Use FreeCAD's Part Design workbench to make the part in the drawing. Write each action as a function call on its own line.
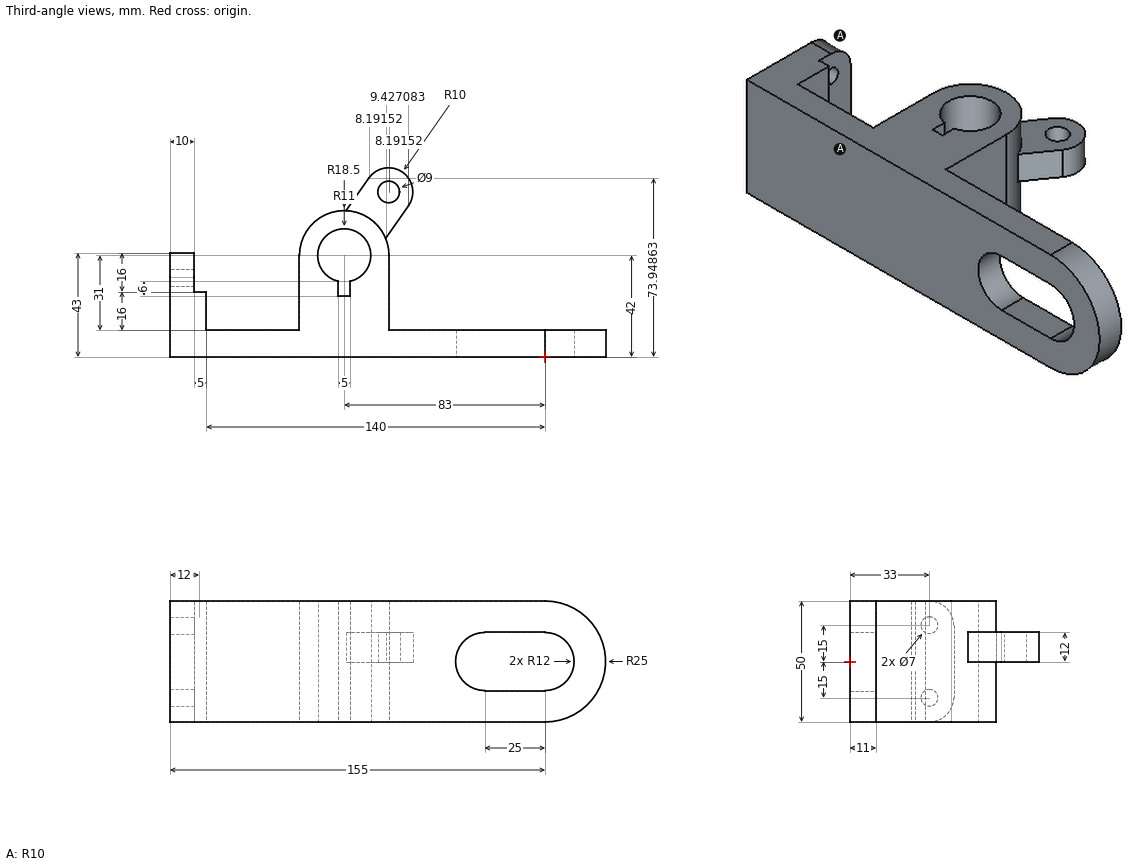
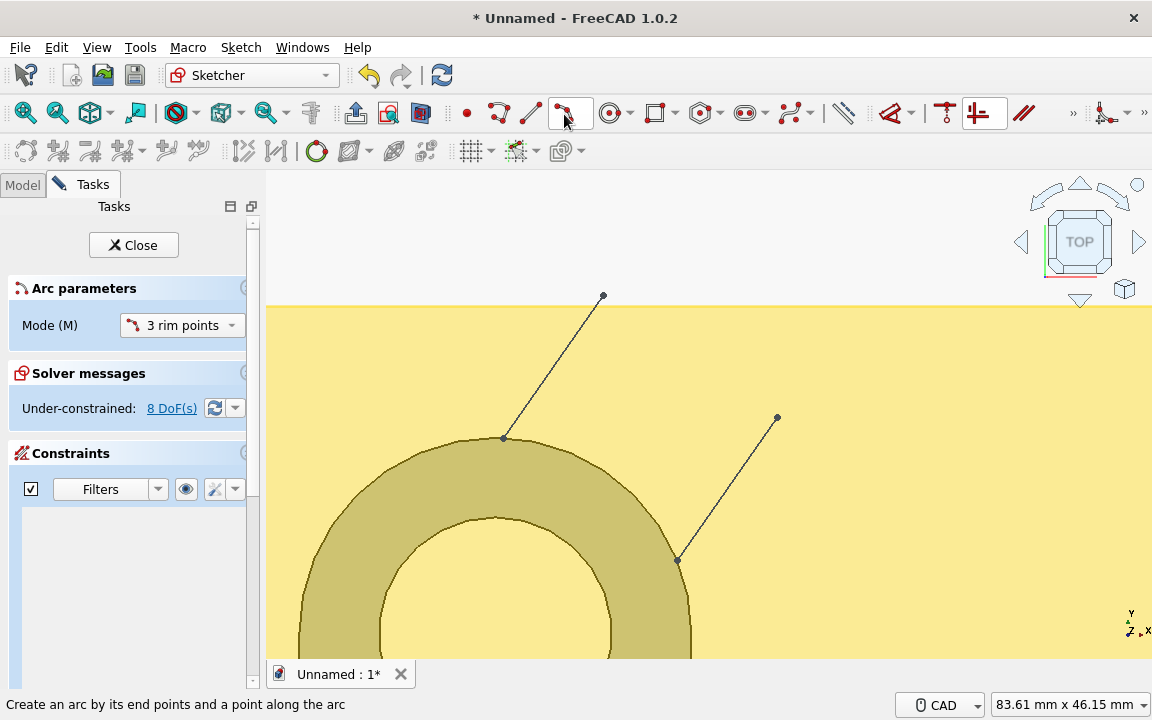
click(777, 418)
click(603, 296)
click(751, 269)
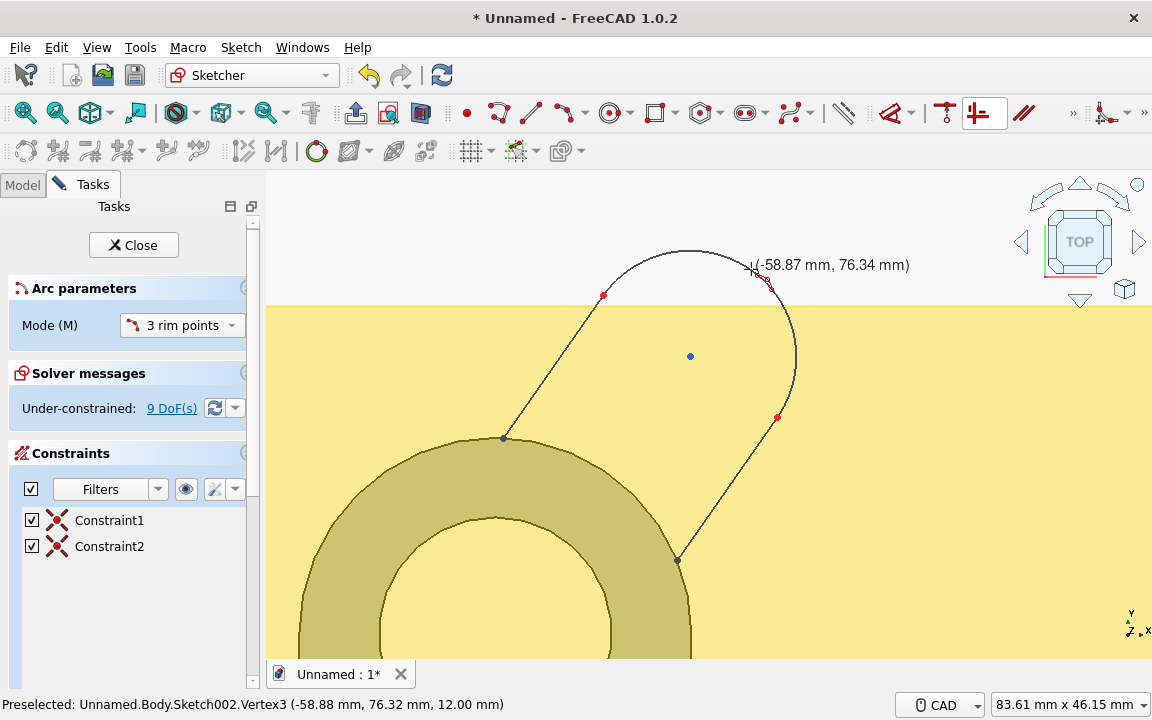
click(503, 439)
click(677, 561)
click(608, 473)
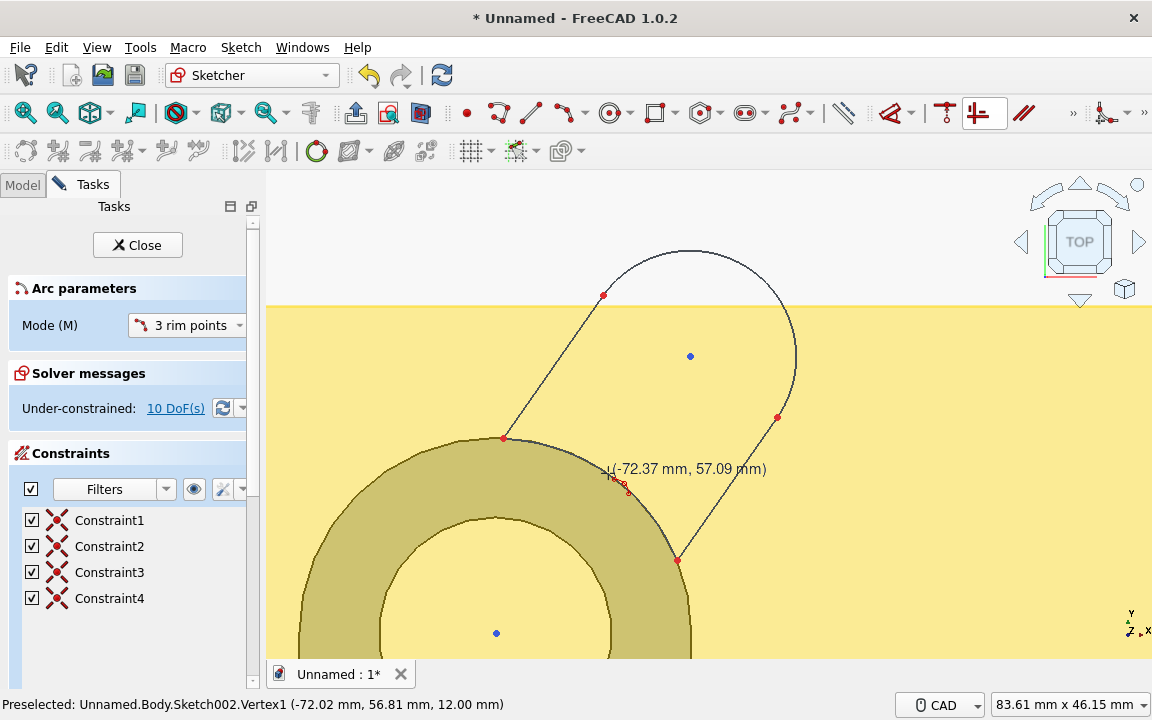
click(610, 114)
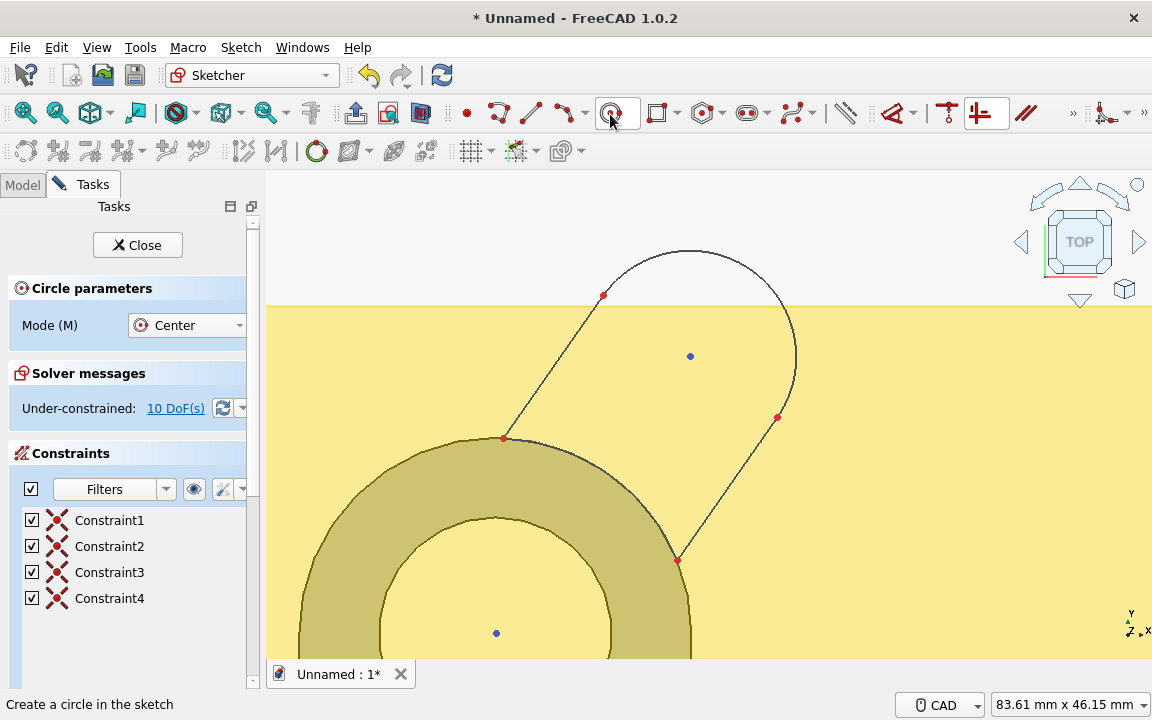
click(690, 356)
move(724, 322)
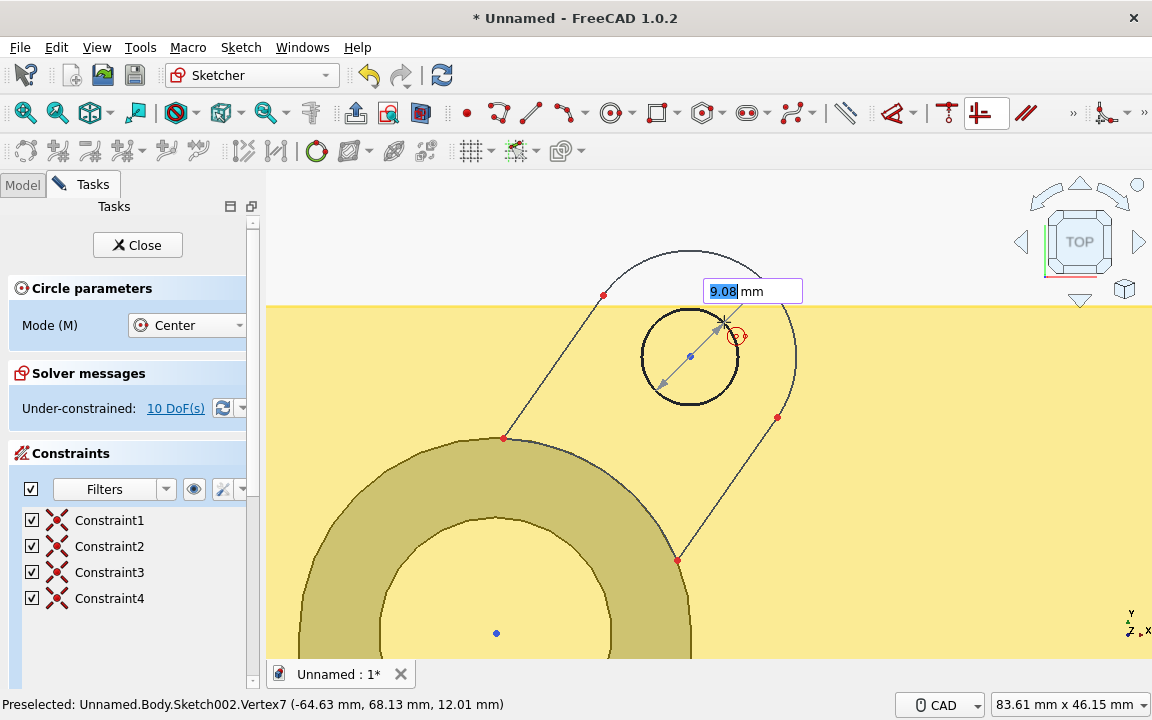
text(9)
key(Return)
key(Escape)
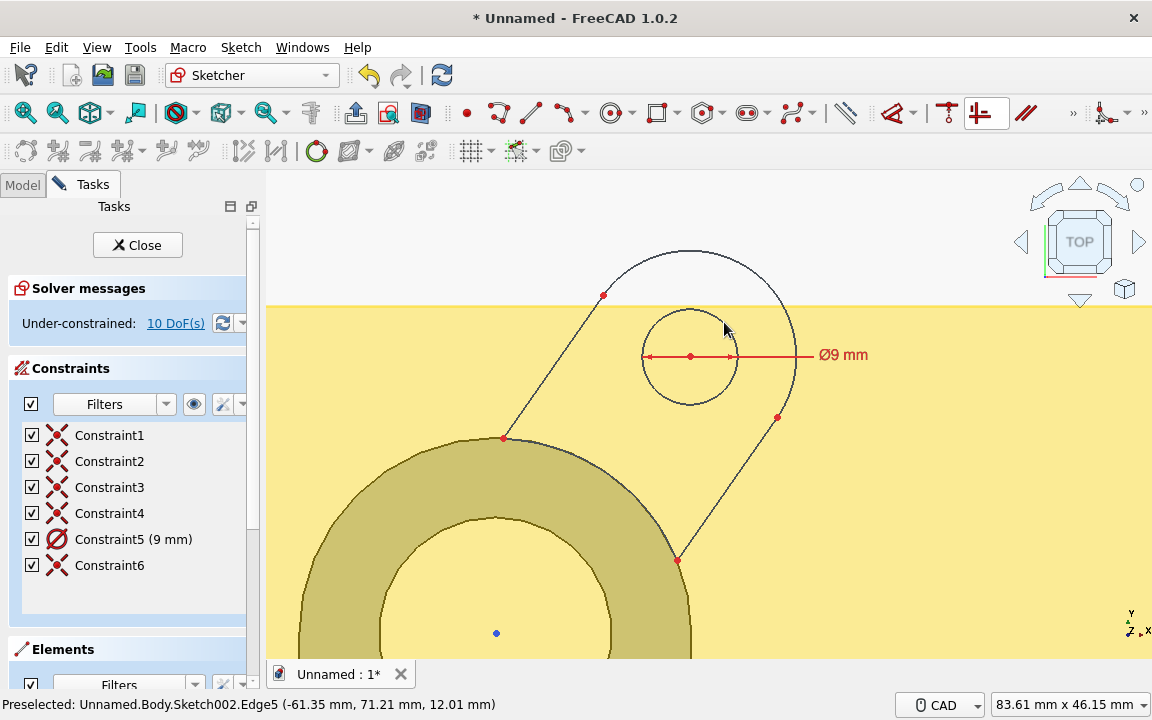
click(707, 518)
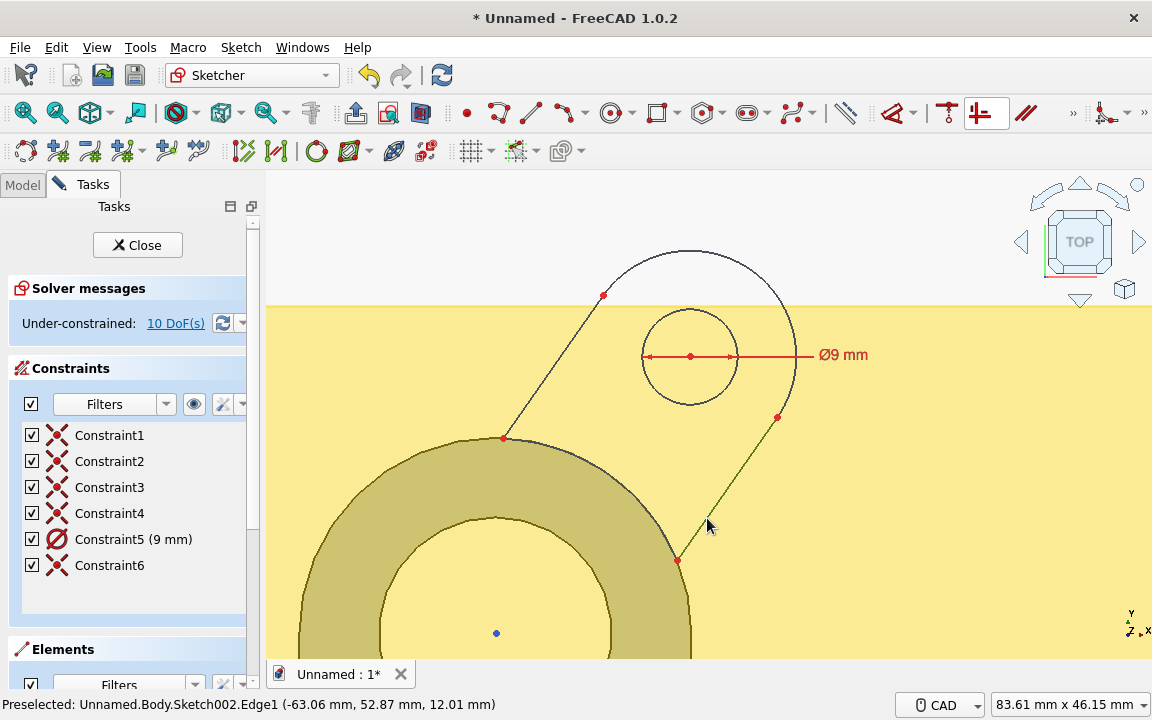
click(790, 322)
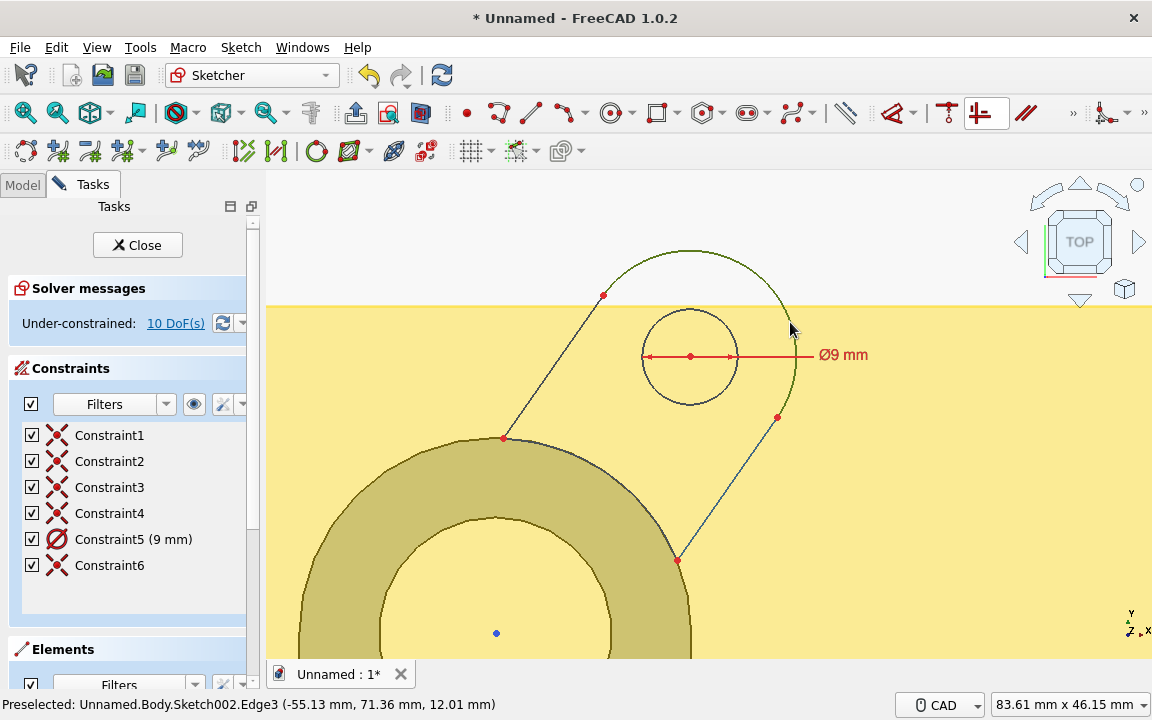
key(t)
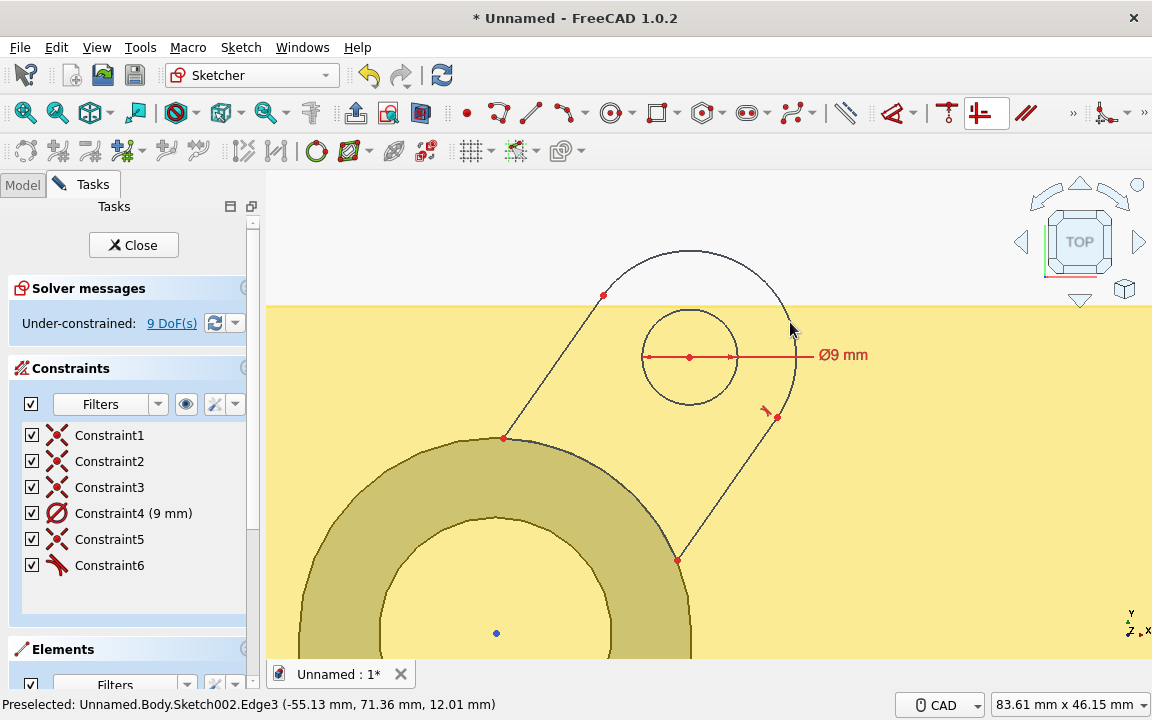
click(573, 339)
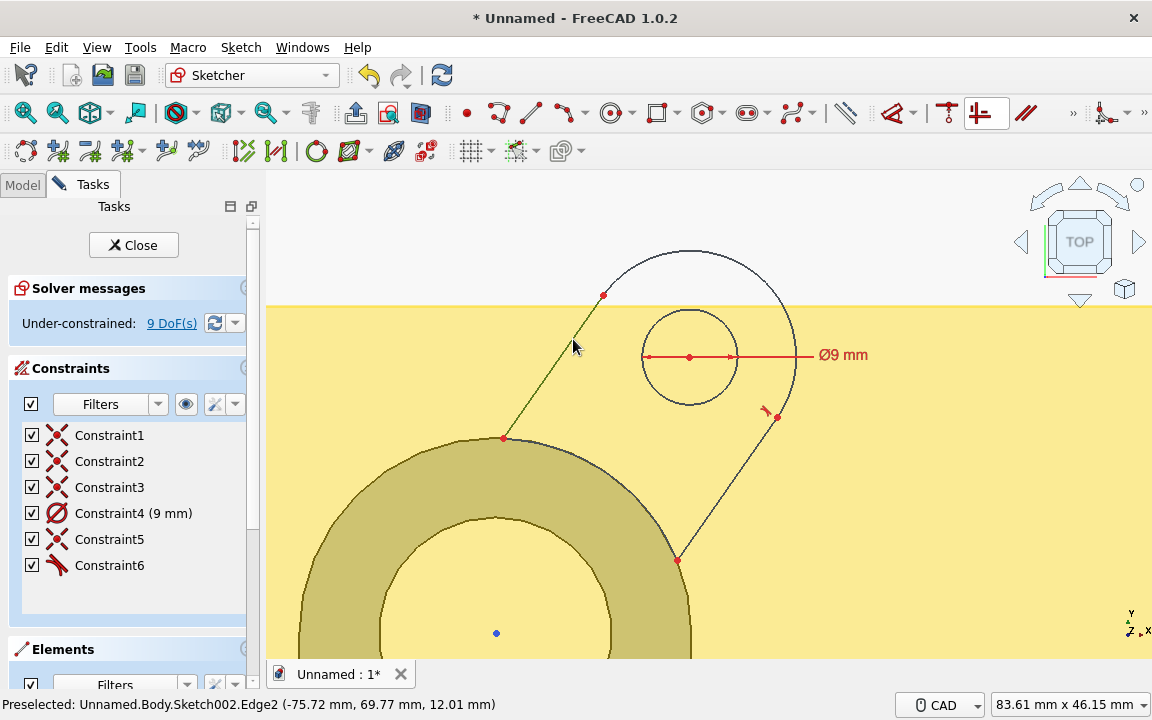
click(790, 323)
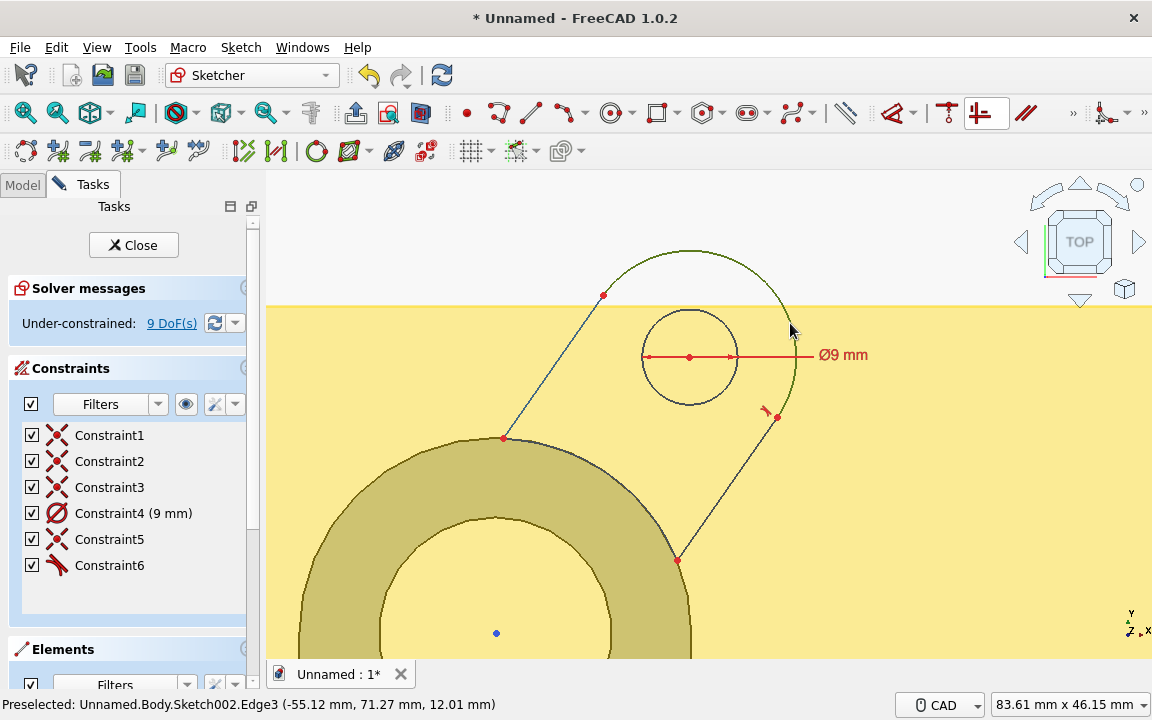
key(t)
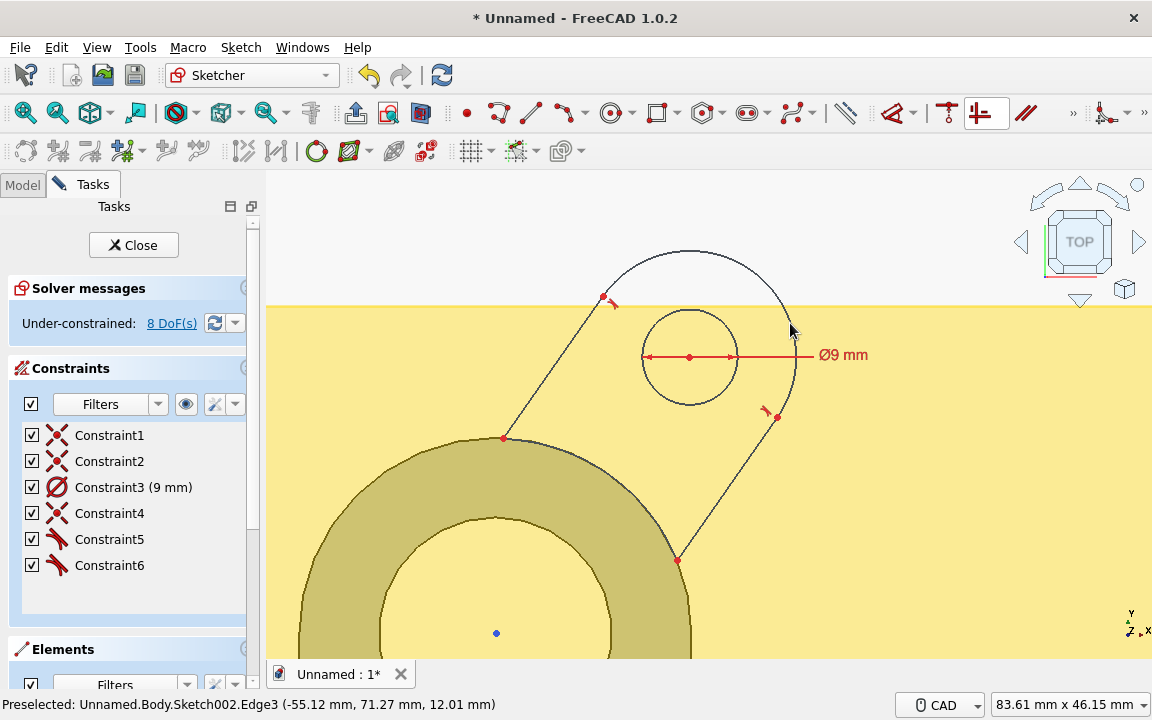
click(892, 114)